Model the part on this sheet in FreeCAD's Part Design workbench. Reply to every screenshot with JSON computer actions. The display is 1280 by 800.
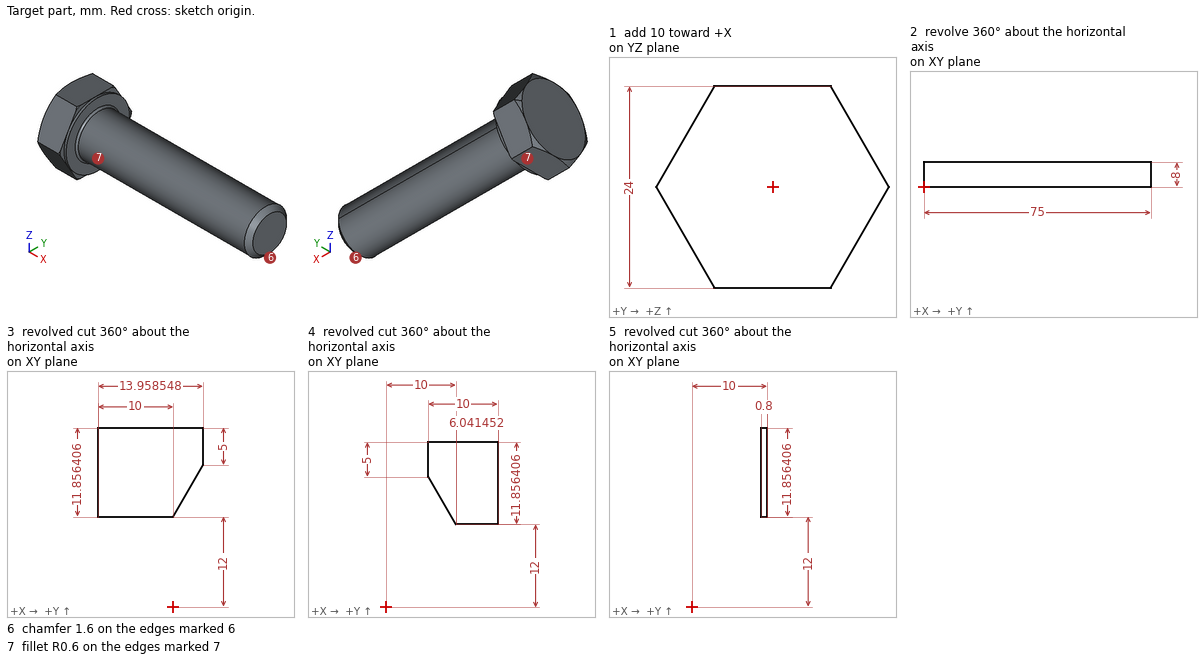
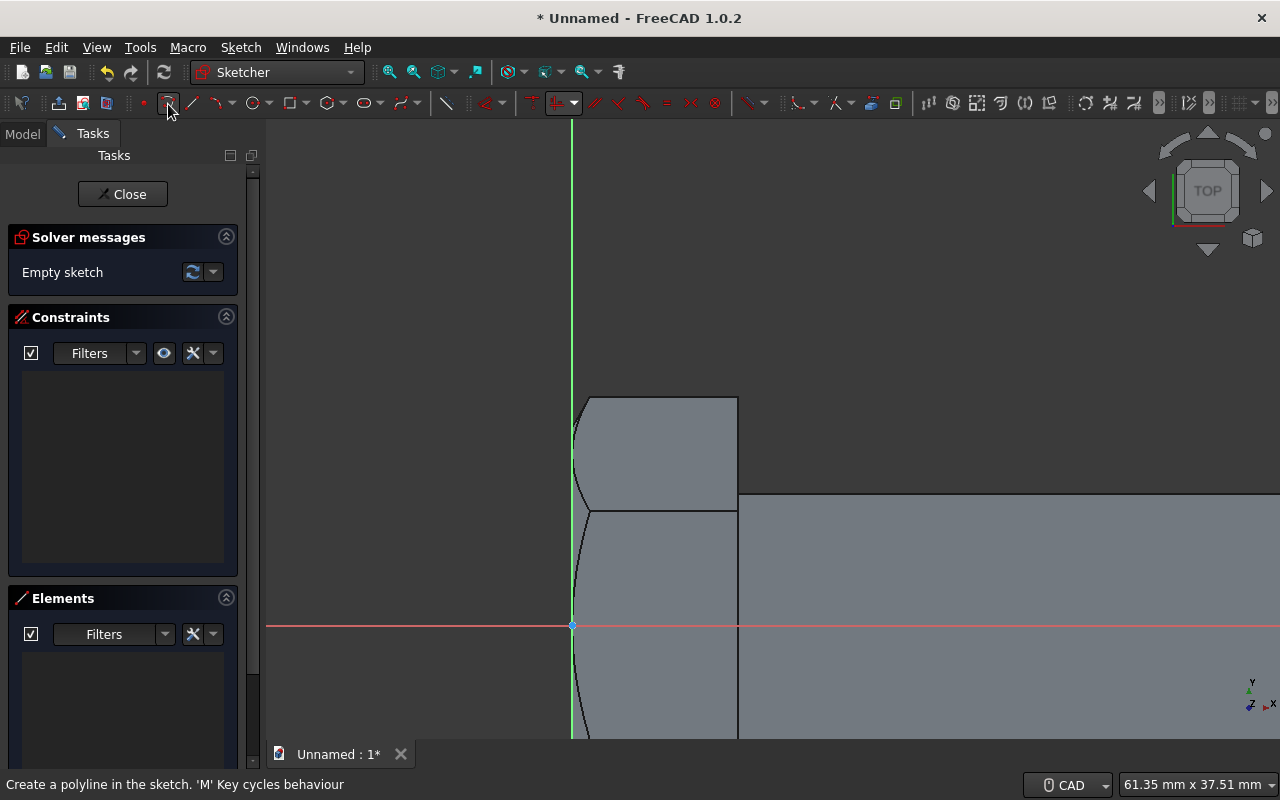
{"action": "left_click", "coordinate": [738, 427]}
{"action": "left_click", "coordinate": [837, 427]}
{"action": "left_click", "coordinate": [837, 231]}
{"action": "left_click", "coordinate": [672, 231]}
{"action": "left_click", "coordinate": [672, 314]}
{"action": "left_click", "coordinate": [738, 428]}
{"action": "key", "text": "Escape"}
{"action": "key", "text": "Escape"}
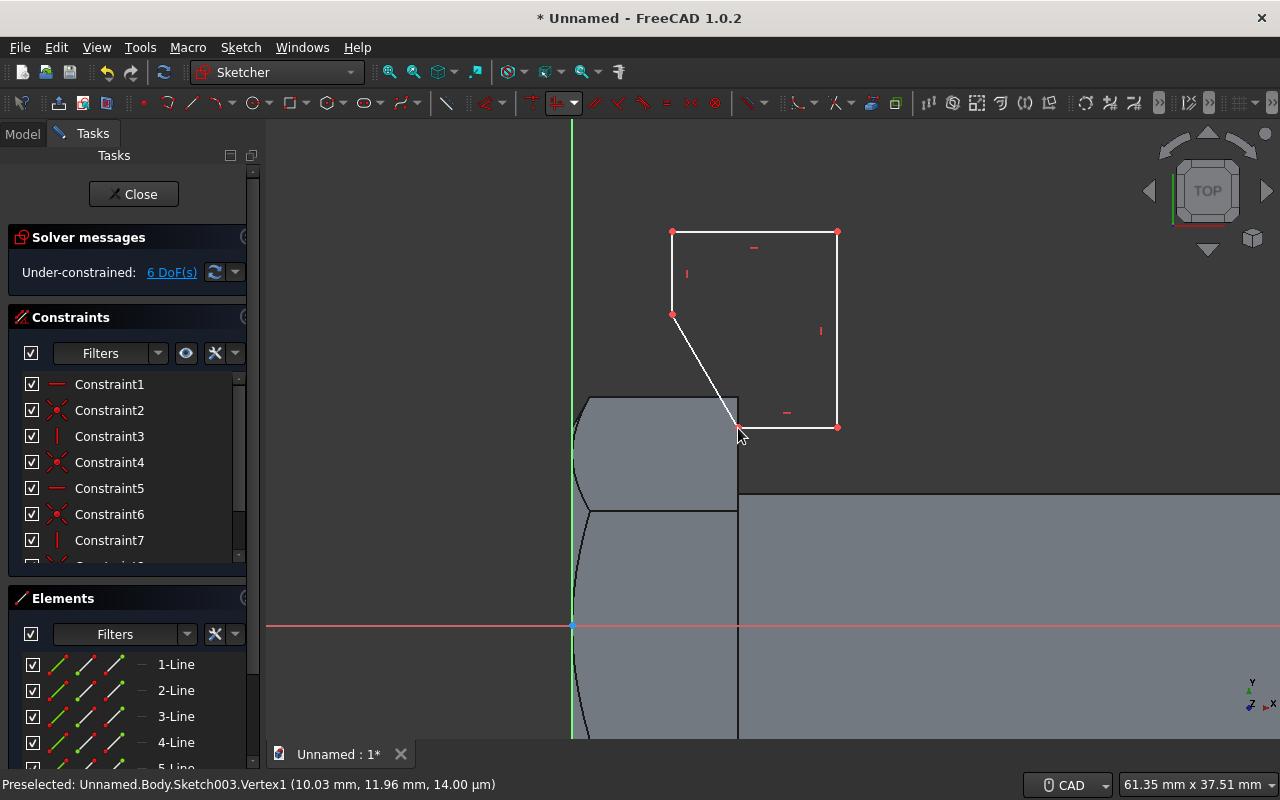
{"action": "left_click", "coordinate": [486, 104]}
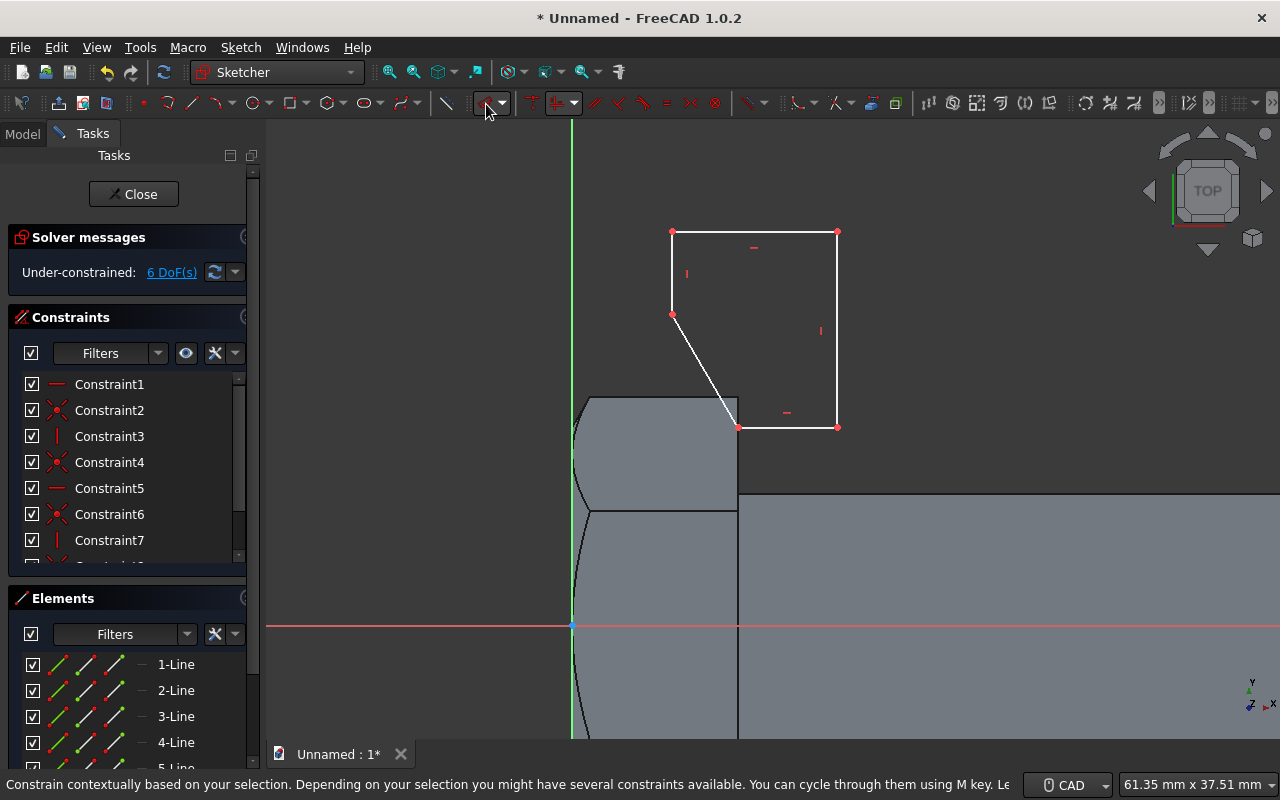
{"action": "left_click", "coordinate": [672, 257]}
{"action": "left_click", "coordinate": [638, 273]}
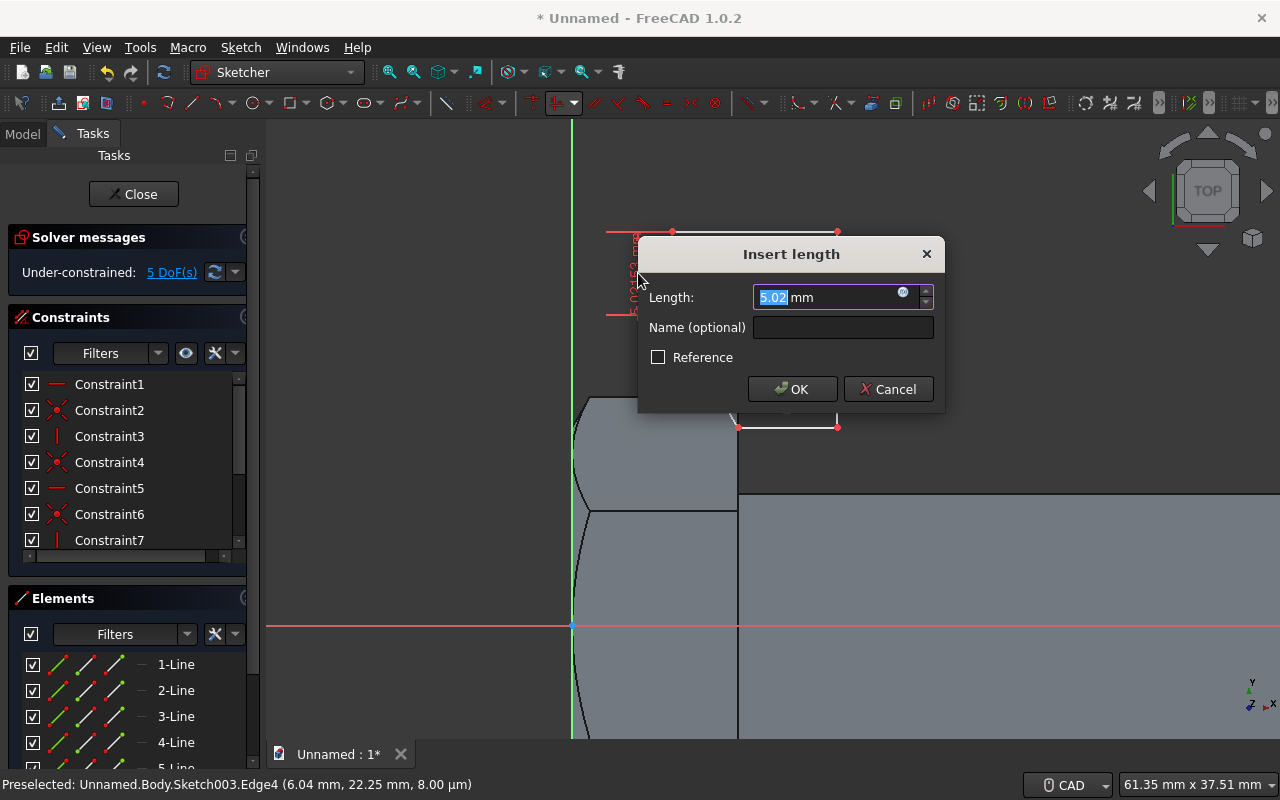
{"action": "type", "text": "5"}
{"action": "key", "text": "Return"}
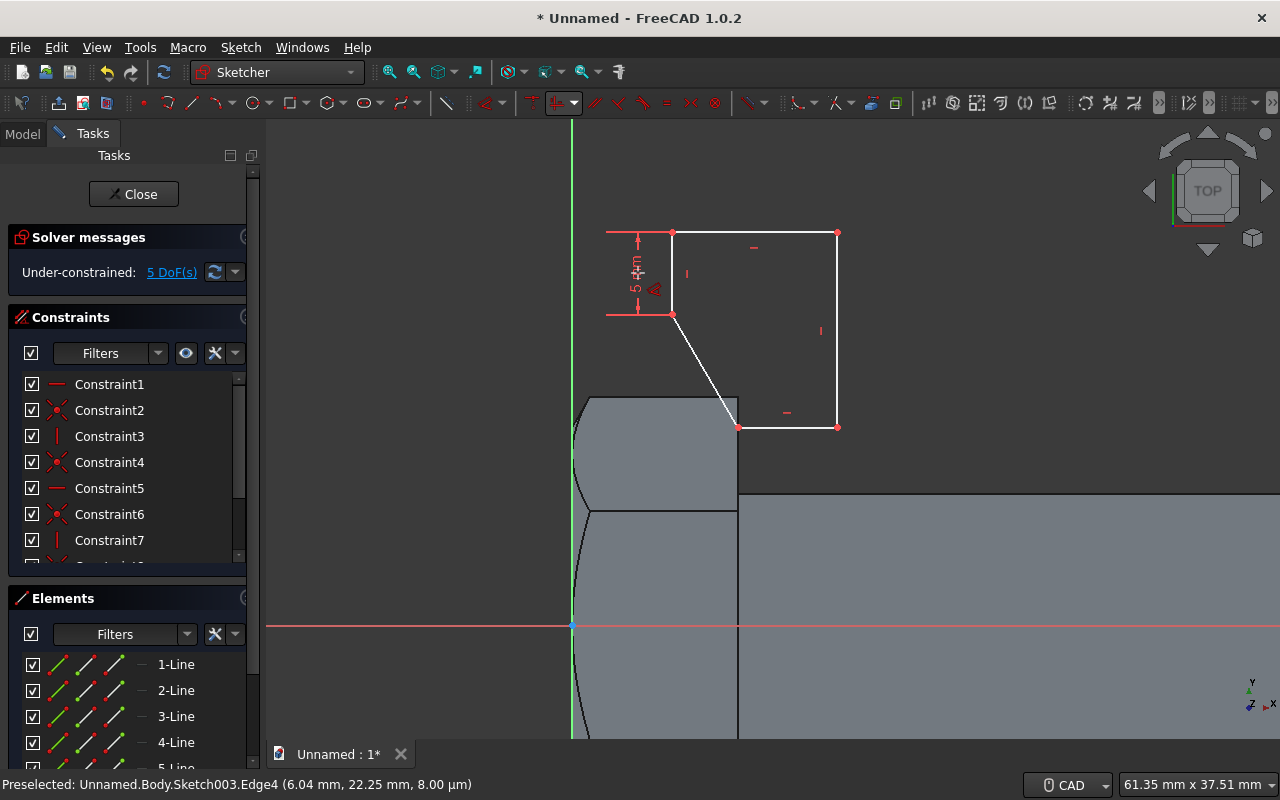
{"action": "left_click", "coordinate": [788, 232]}
{"action": "left_click", "coordinate": [755, 198]}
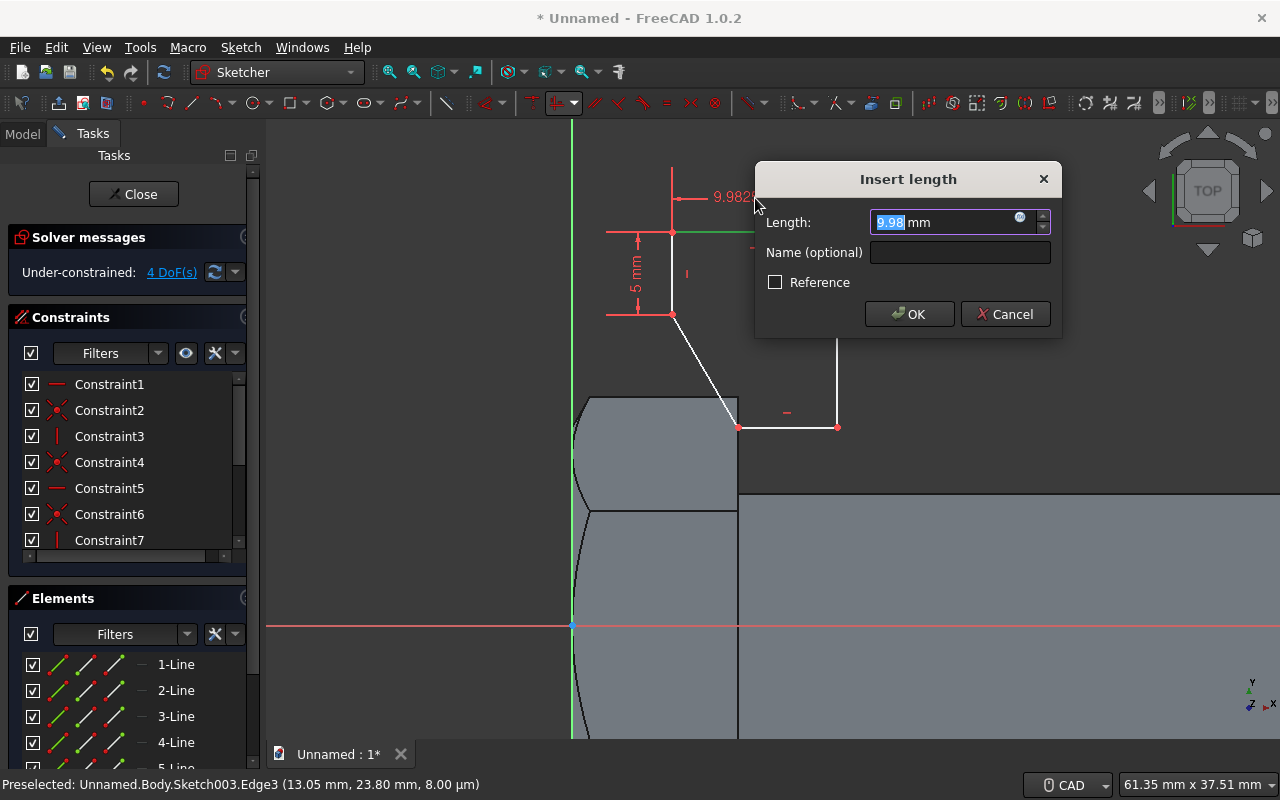
{"action": "type", "text": "10"}
{"action": "key", "text": "Return"}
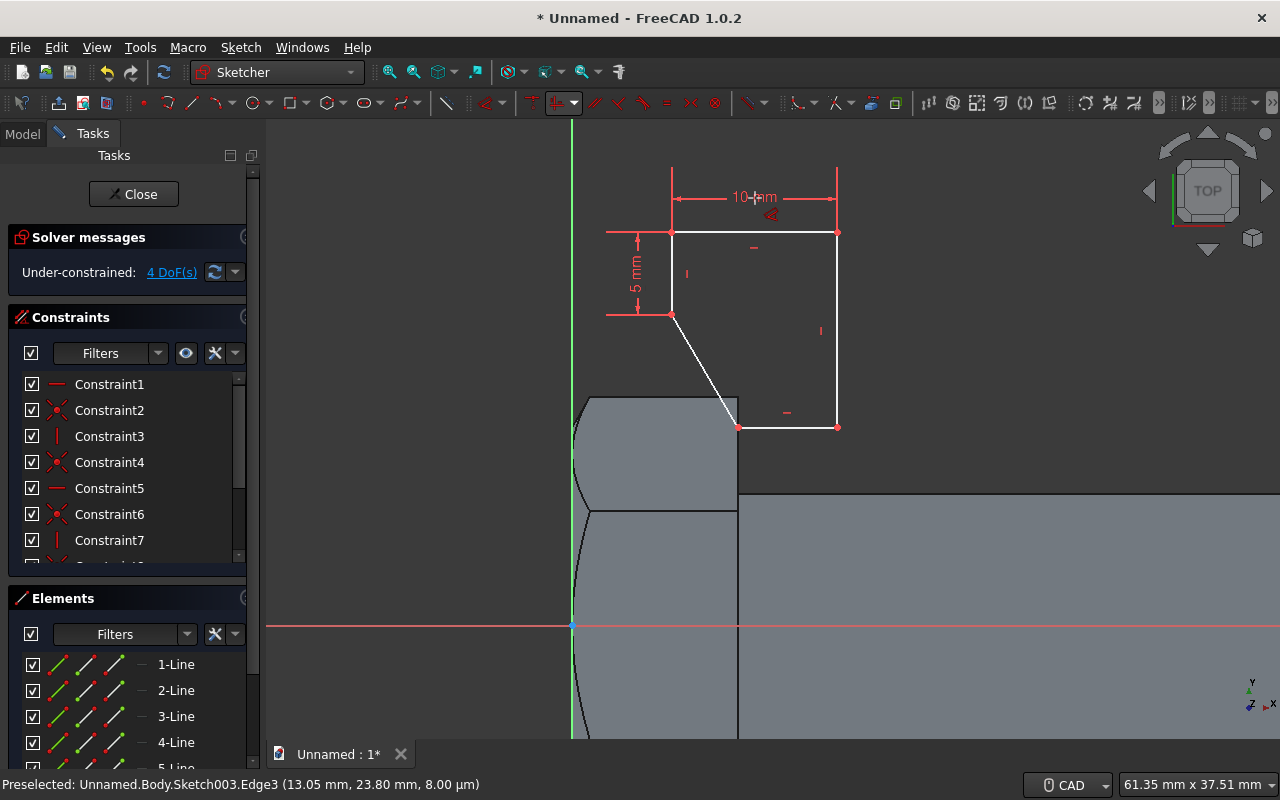
{"action": "left_click", "coordinate": [738, 428]}
{"action": "left_click", "coordinate": [655, 660]}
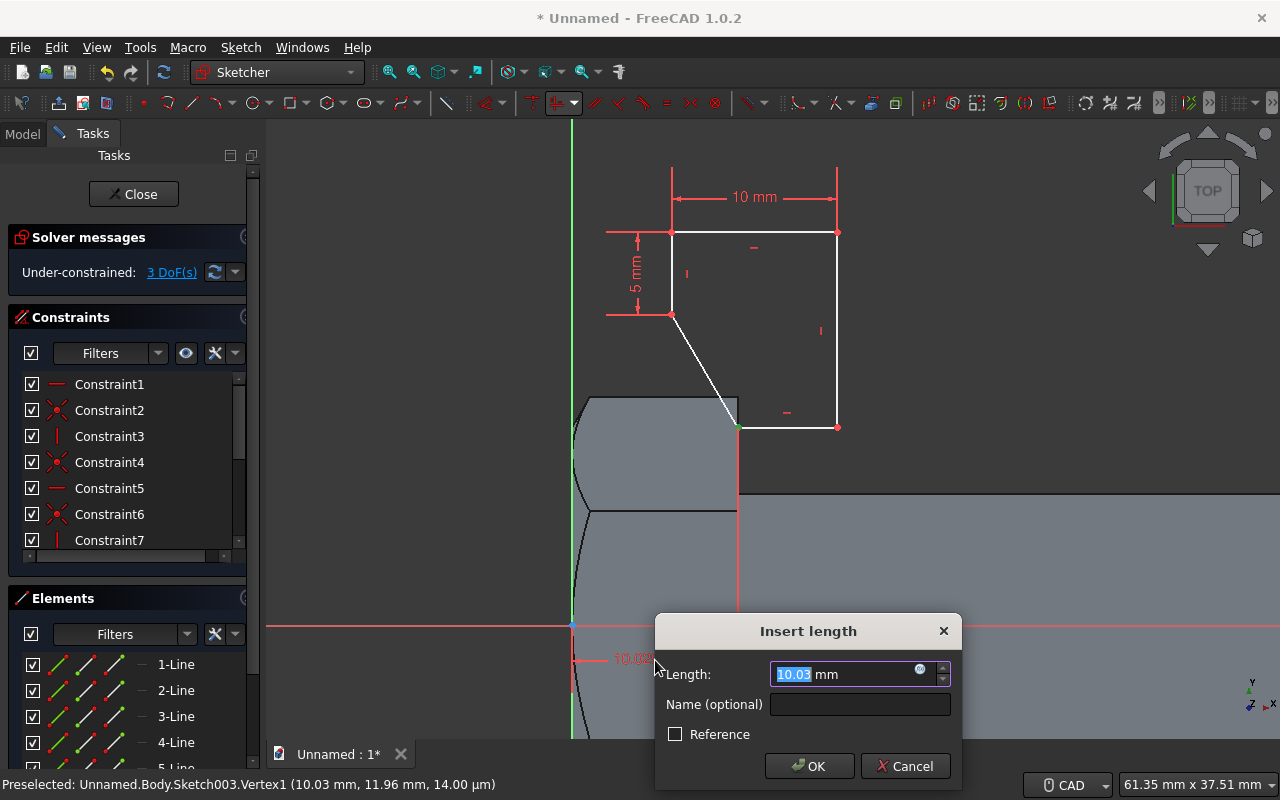
{"action": "type", "text": "10"}
{"action": "key", "text": "Return"}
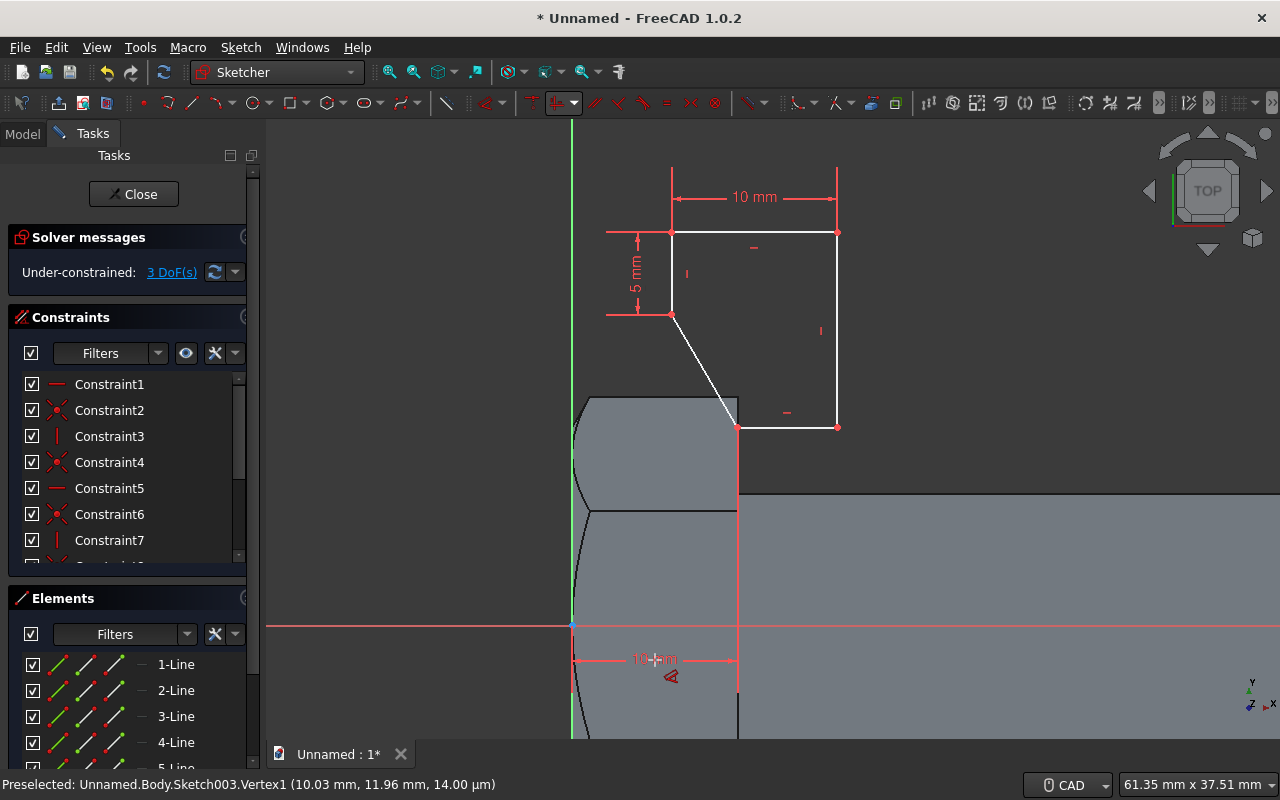
{"action": "left_click", "coordinate": [738, 428]}
{"action": "left_click", "coordinate": [538, 527]}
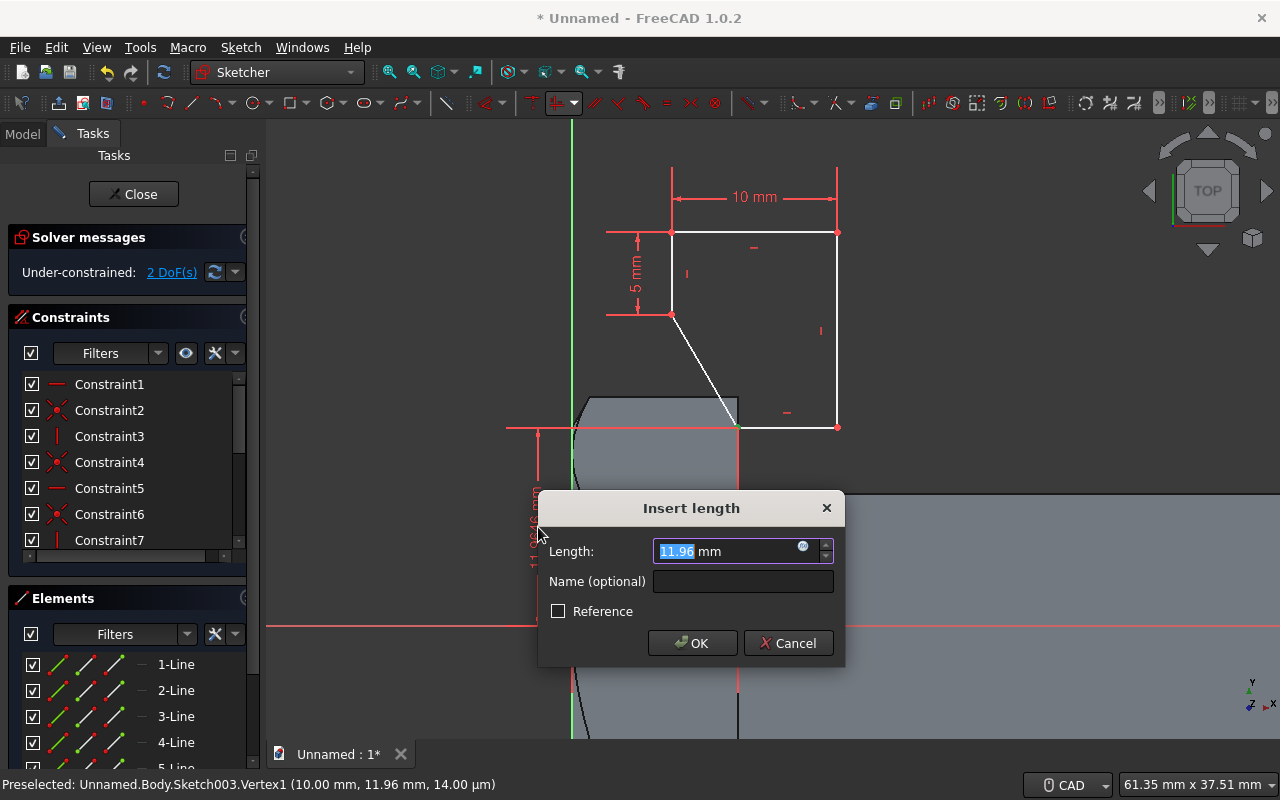
{"action": "type", "text": "12"}
{"action": "key", "text": "Return"}